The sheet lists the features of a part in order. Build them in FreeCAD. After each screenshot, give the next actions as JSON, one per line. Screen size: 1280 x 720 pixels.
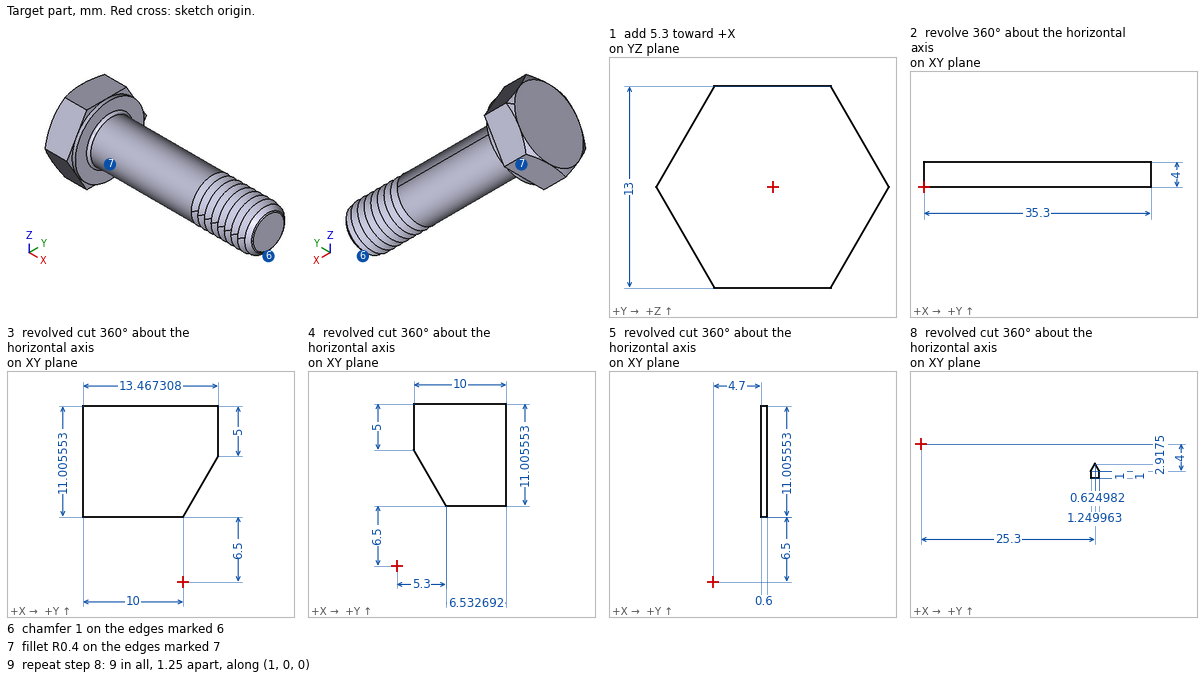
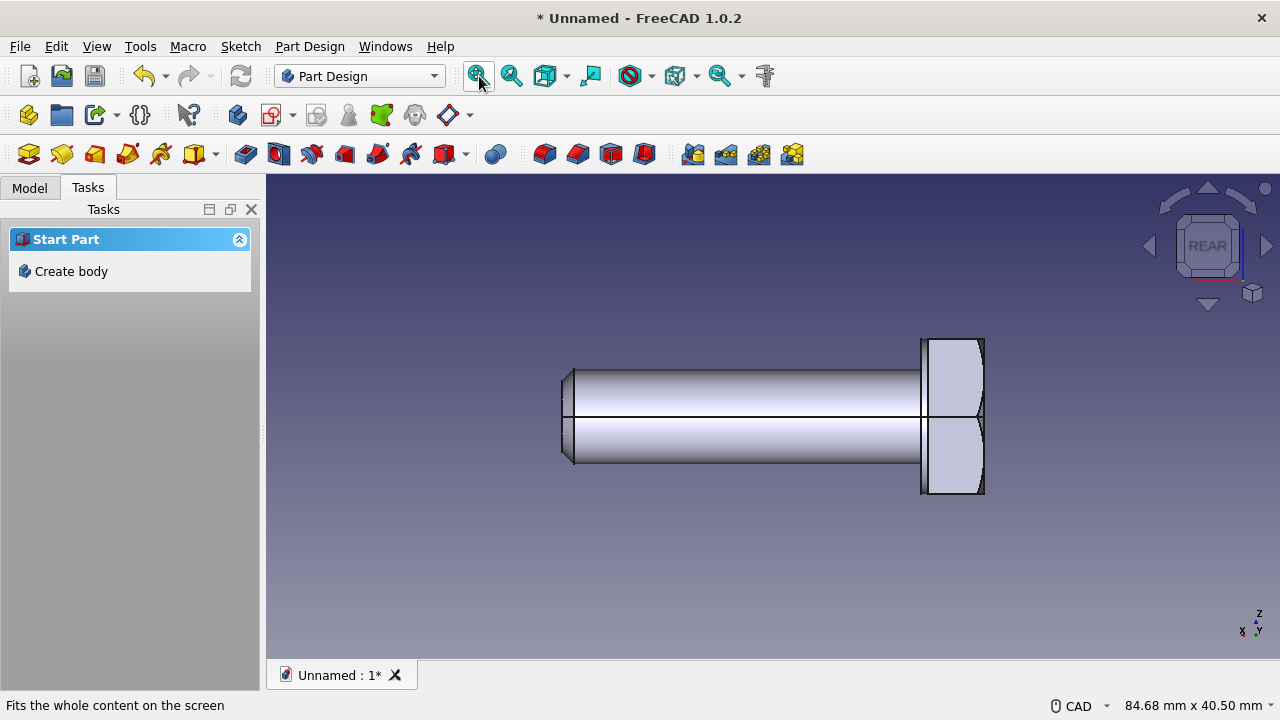
{"action": "key", "text": "6"}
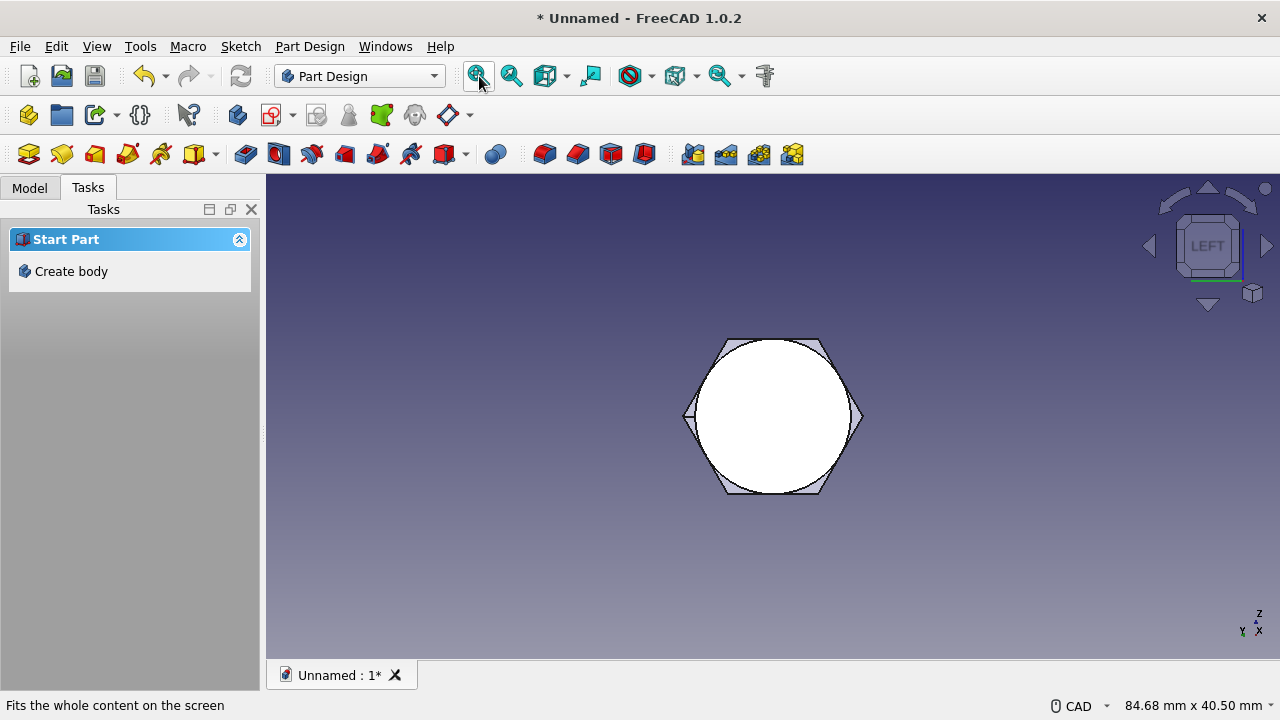
{"action": "left_click", "coordinate": [479, 76]}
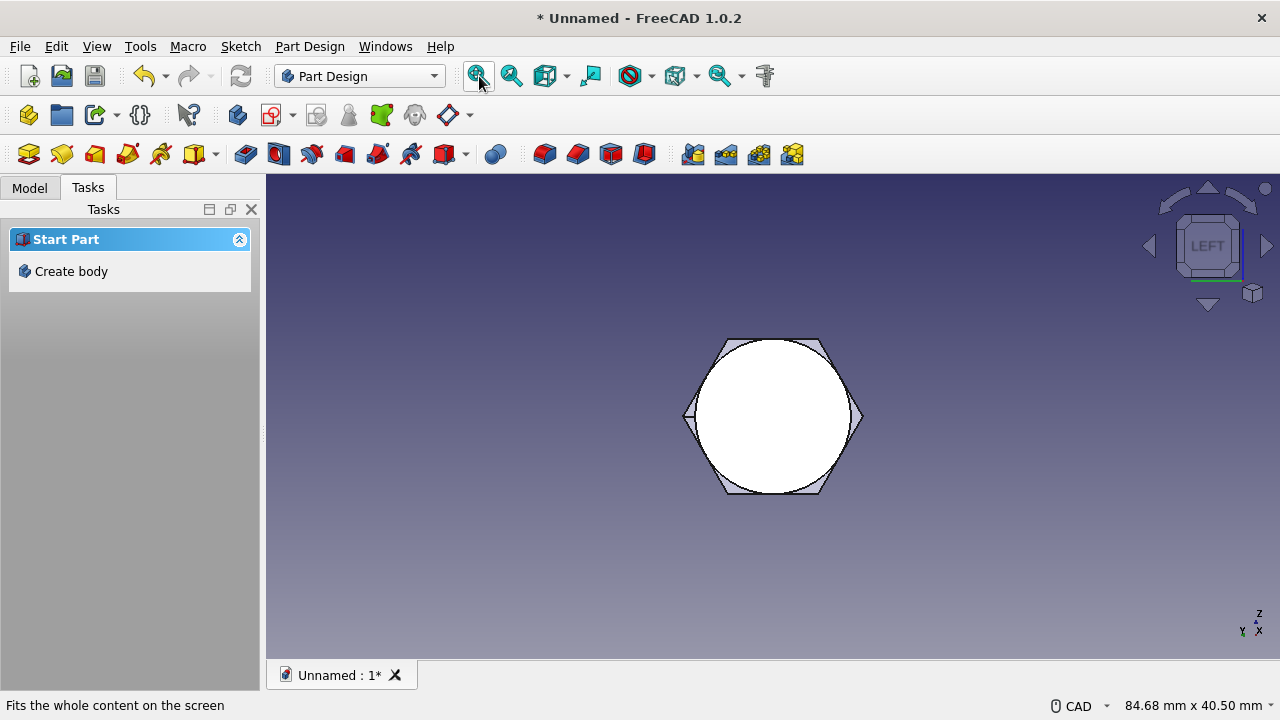
{"action": "key", "text": "v 3"}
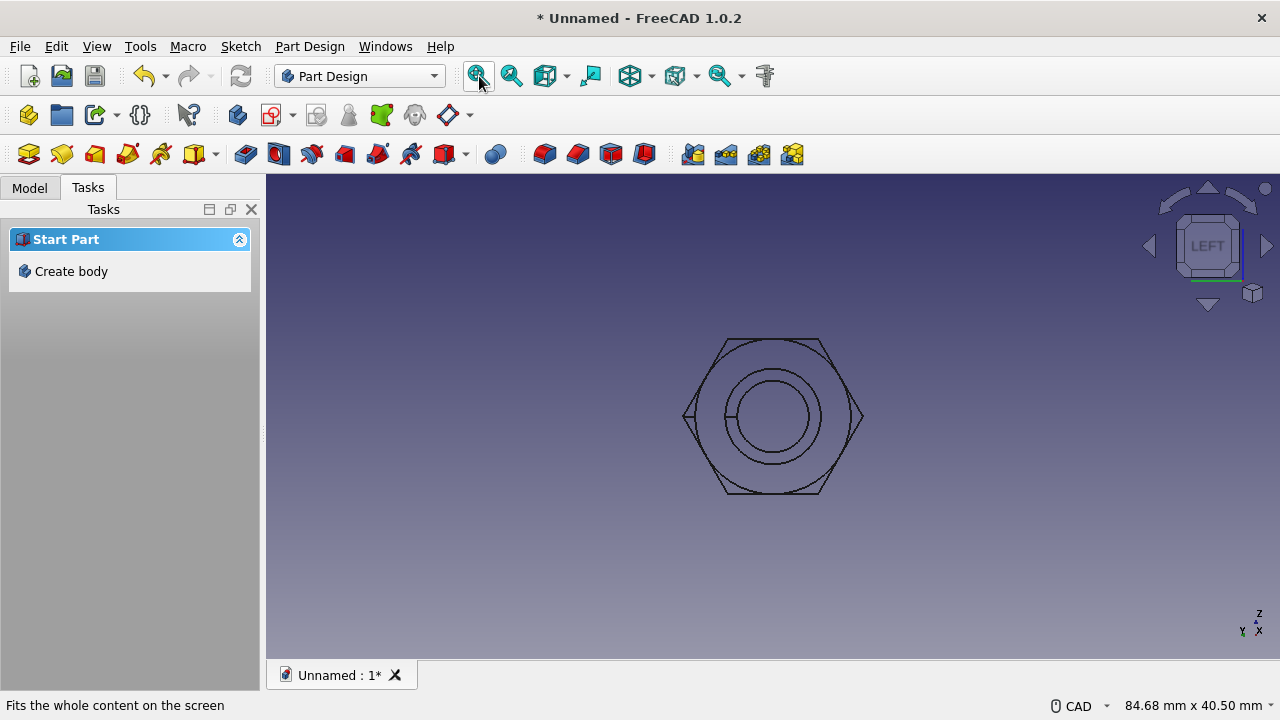
{"action": "key", "text": "0"}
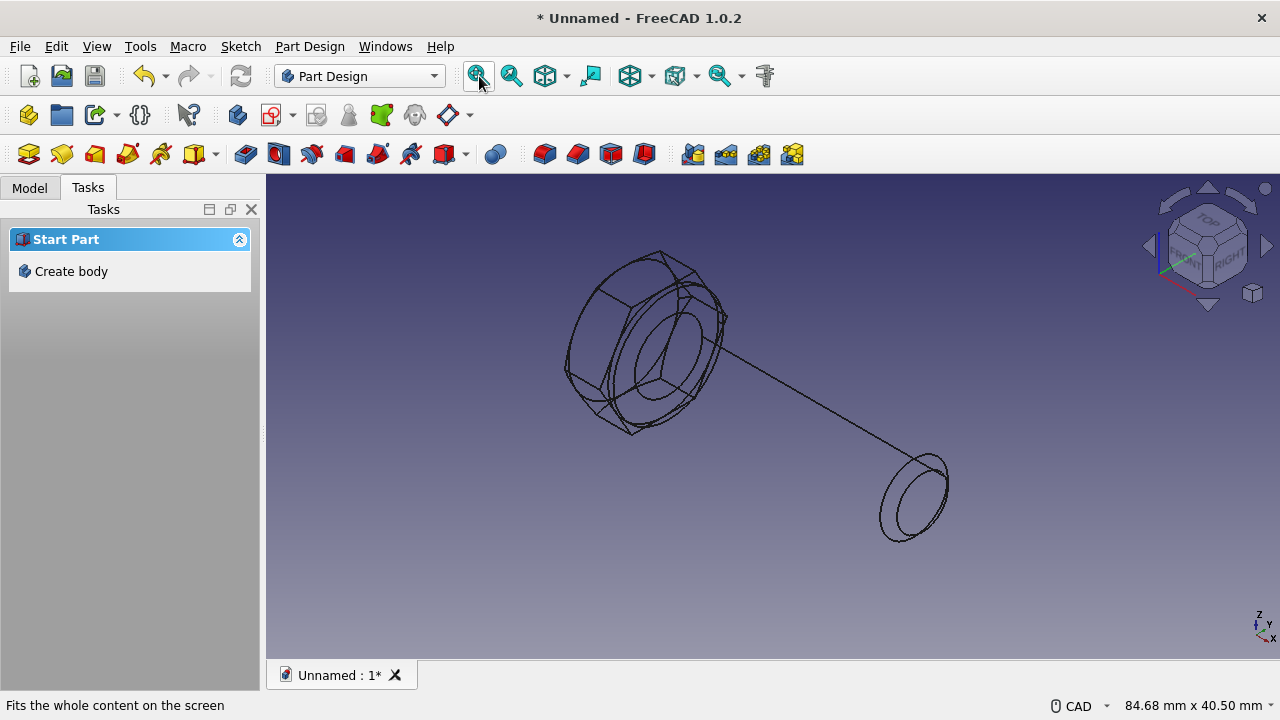
{"action": "left_click", "coordinate": [635, 375]}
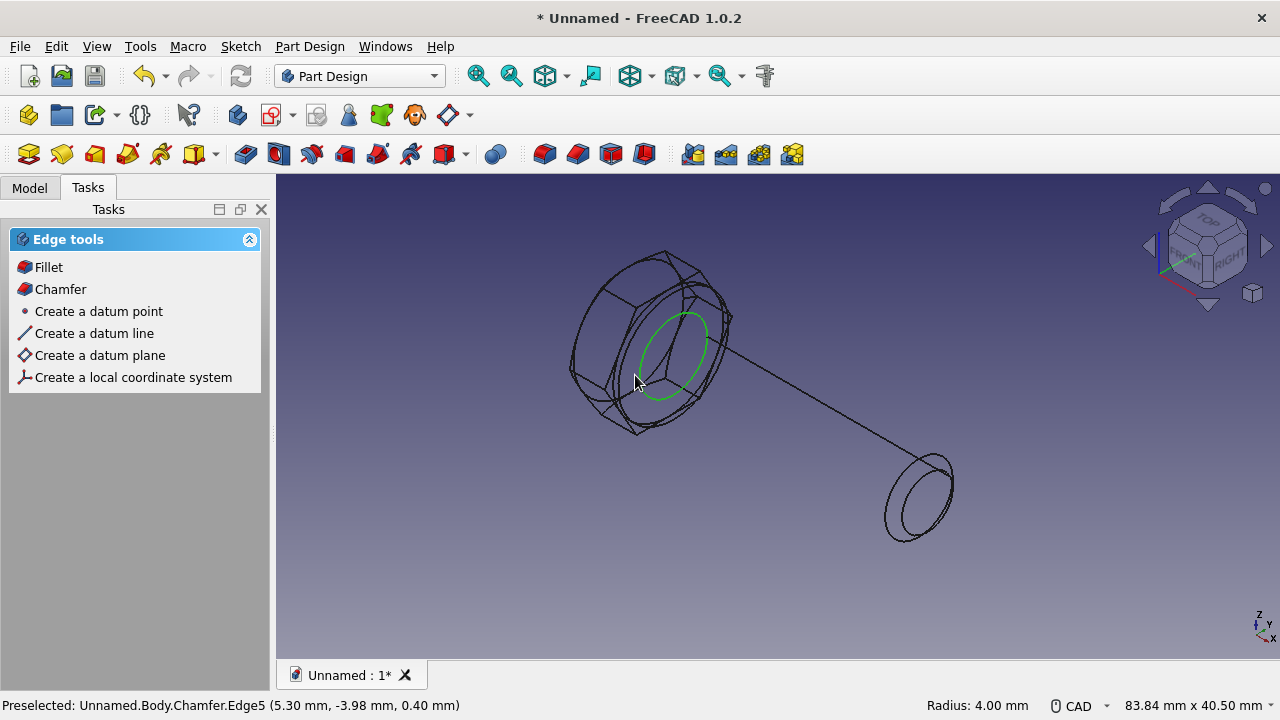
{"action": "key", "text": "v 1"}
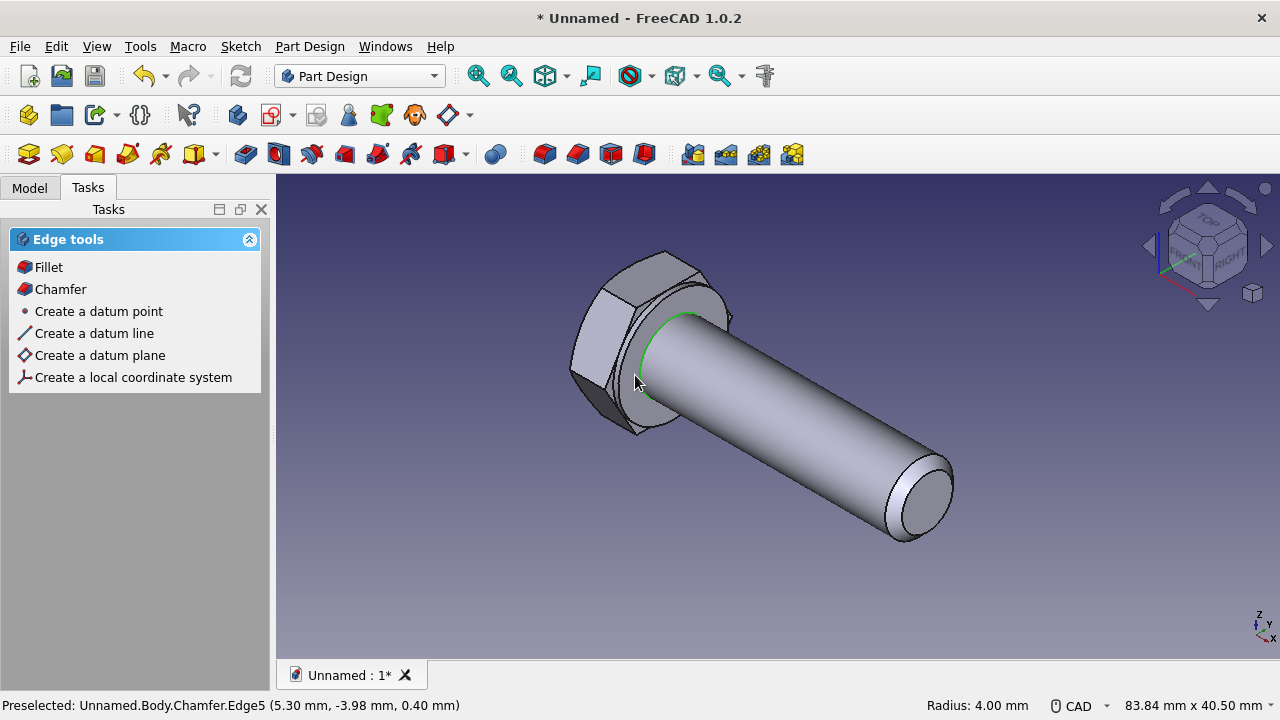
{"action": "left_click", "coordinate": [545, 154]}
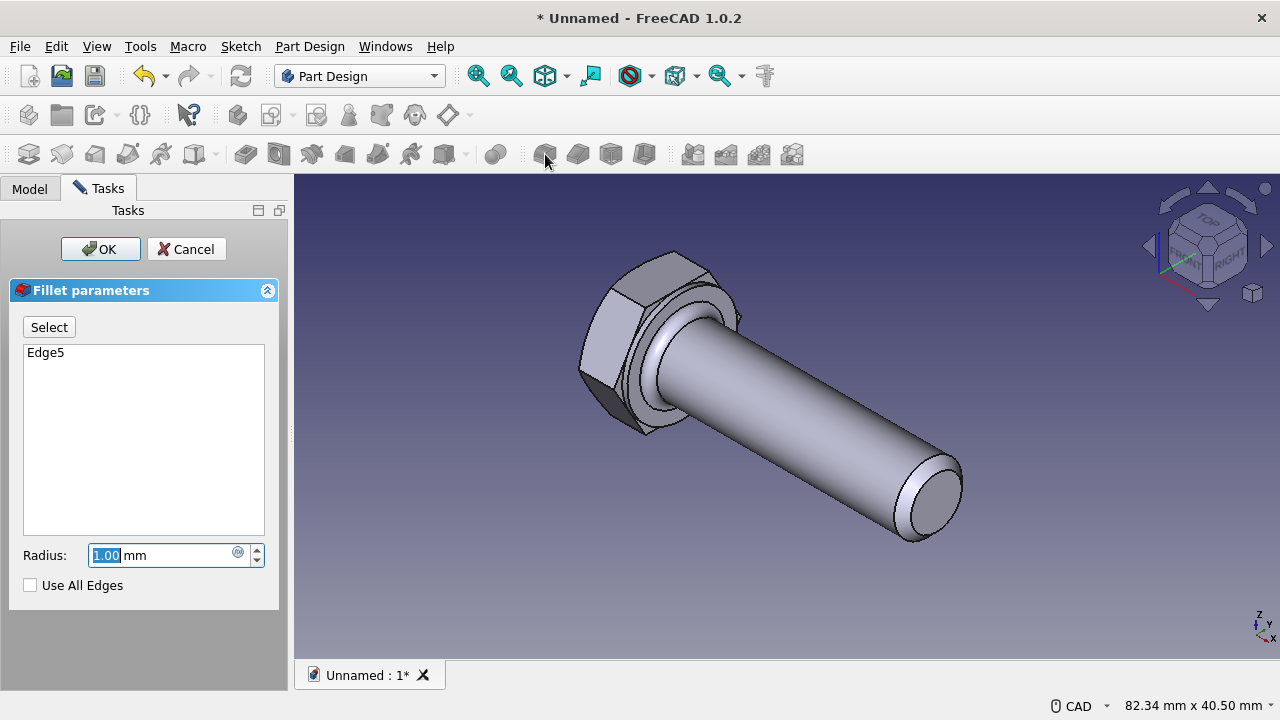
{"action": "type", "text": "0.4"}
{"action": "key", "text": "Tab"}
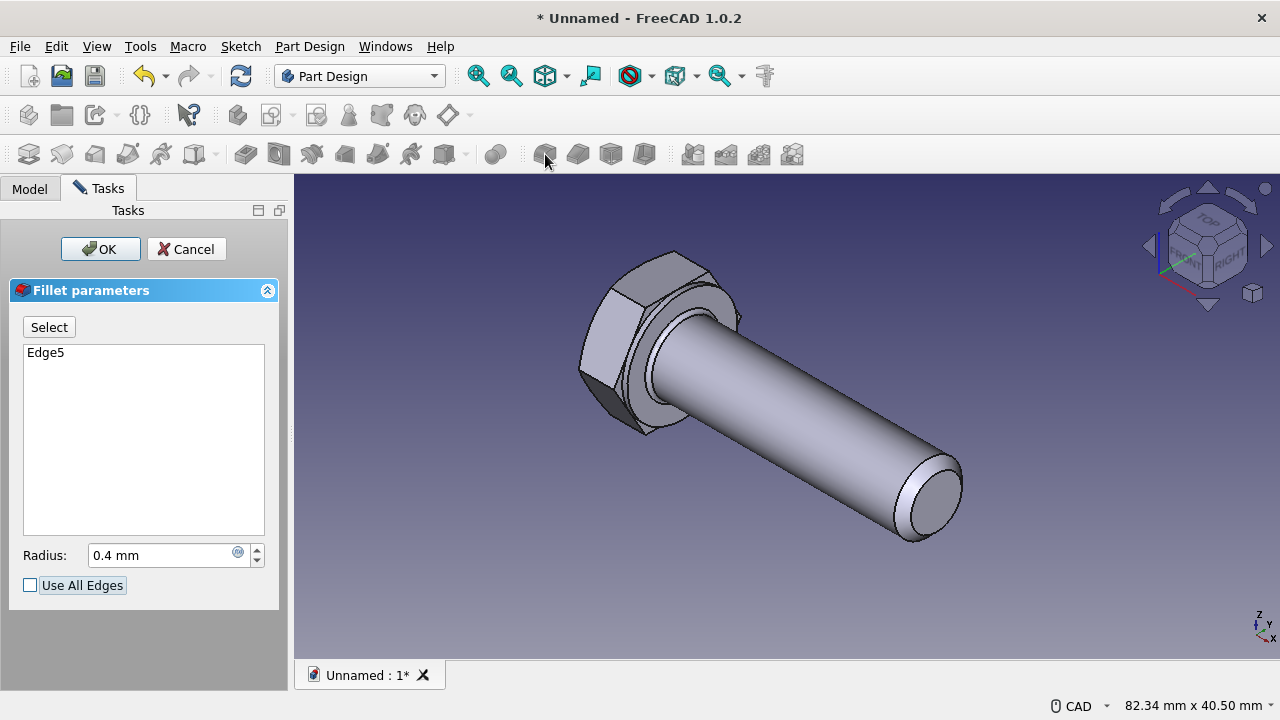
{"action": "left_click", "coordinate": [101, 249]}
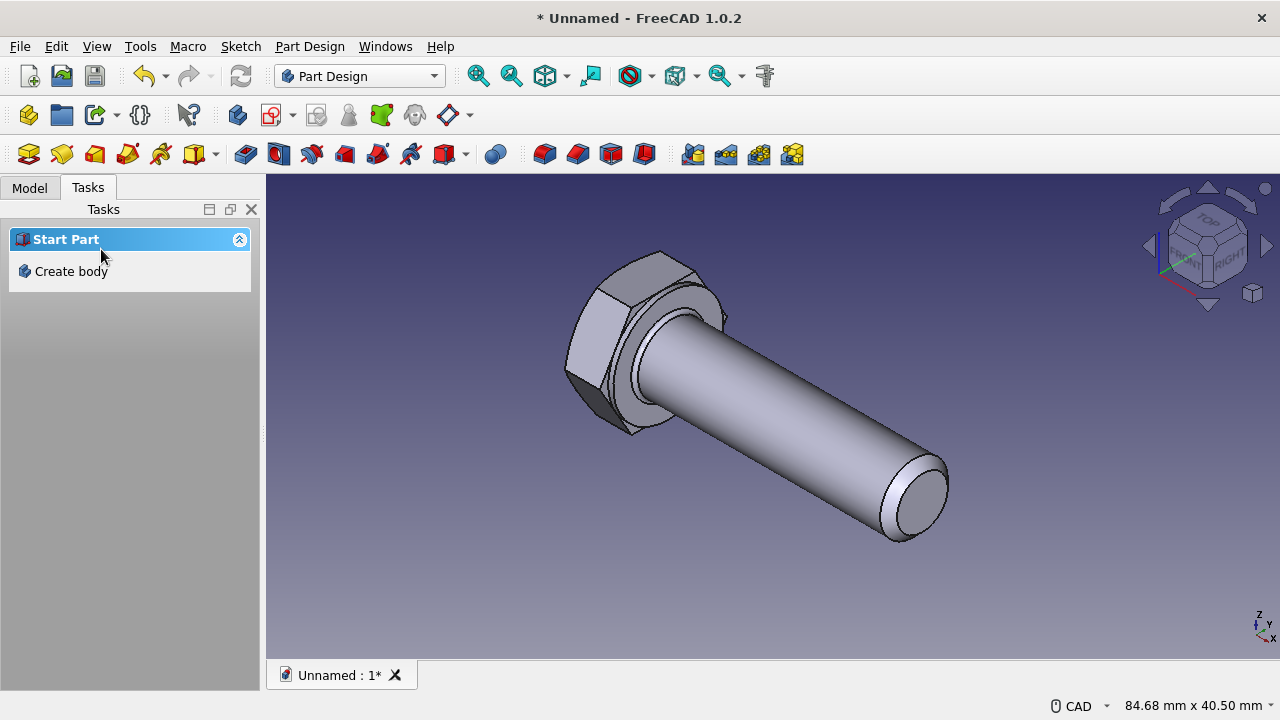
{"action": "left_click", "coordinate": [270, 116]}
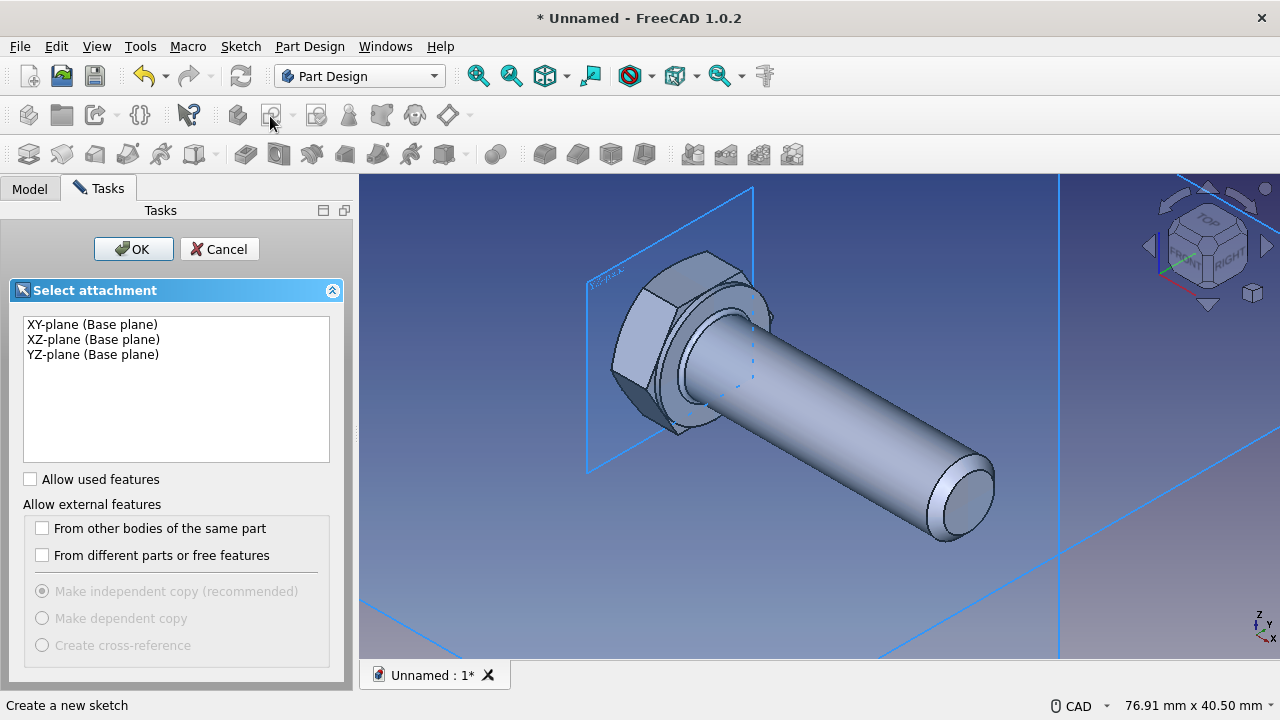
{"action": "left_click", "coordinate": [84, 324]}